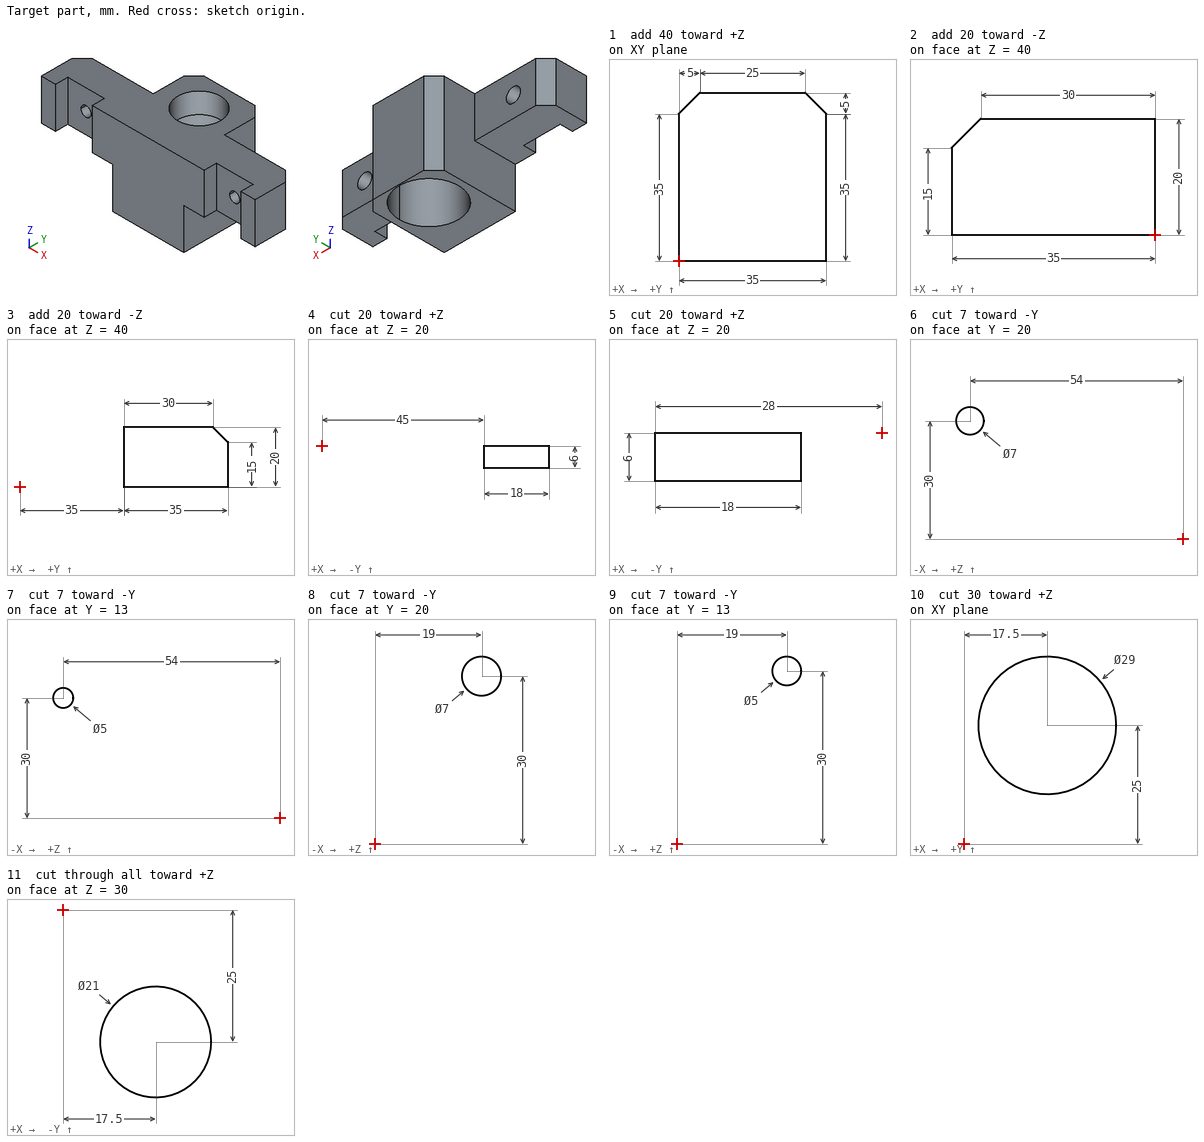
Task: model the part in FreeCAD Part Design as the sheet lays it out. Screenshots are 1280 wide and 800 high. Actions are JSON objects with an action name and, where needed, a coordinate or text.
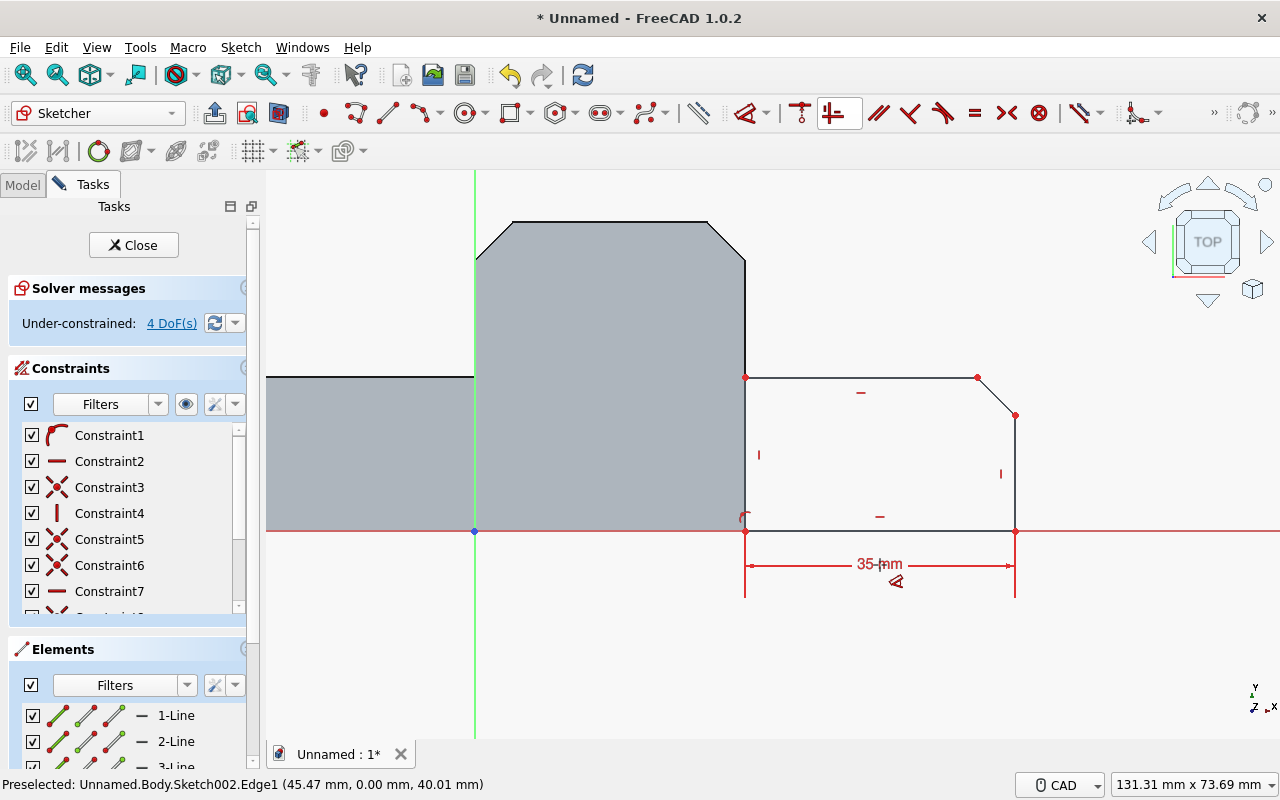
{"action": "left_click", "coordinate": [1015, 497]}
{"action": "left_click", "coordinate": [1049, 474]}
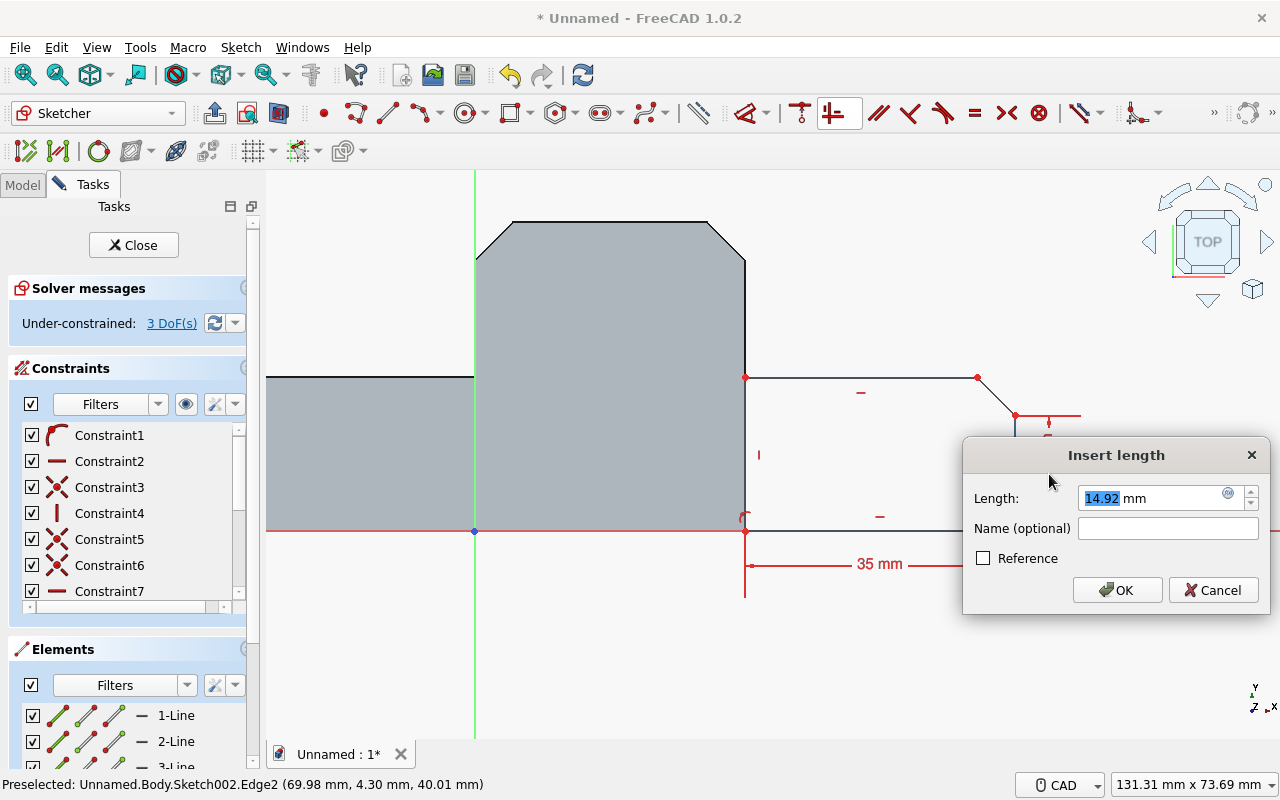
{"action": "type", "text": "15"}
{"action": "key", "text": "Return"}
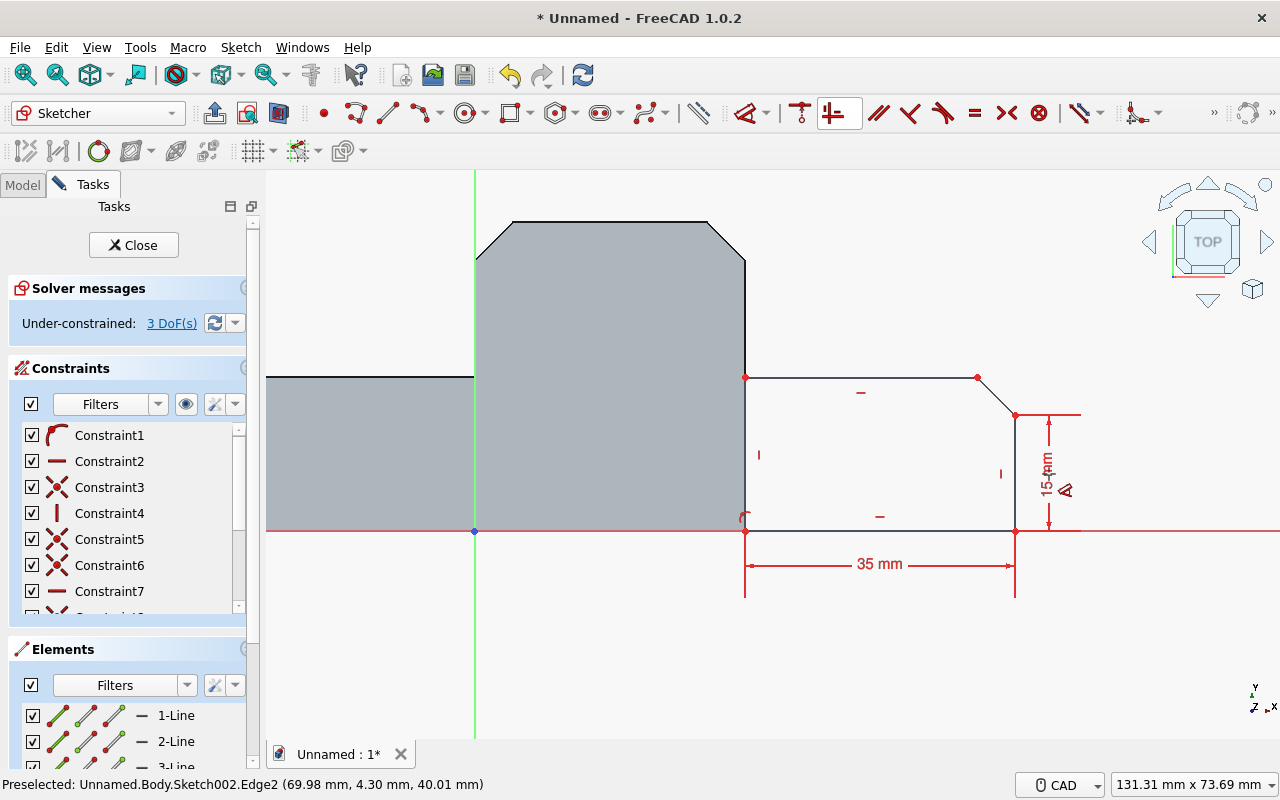
{"action": "left_click", "coordinate": [907, 378]}
{"action": "left_click", "coordinate": [861, 344]}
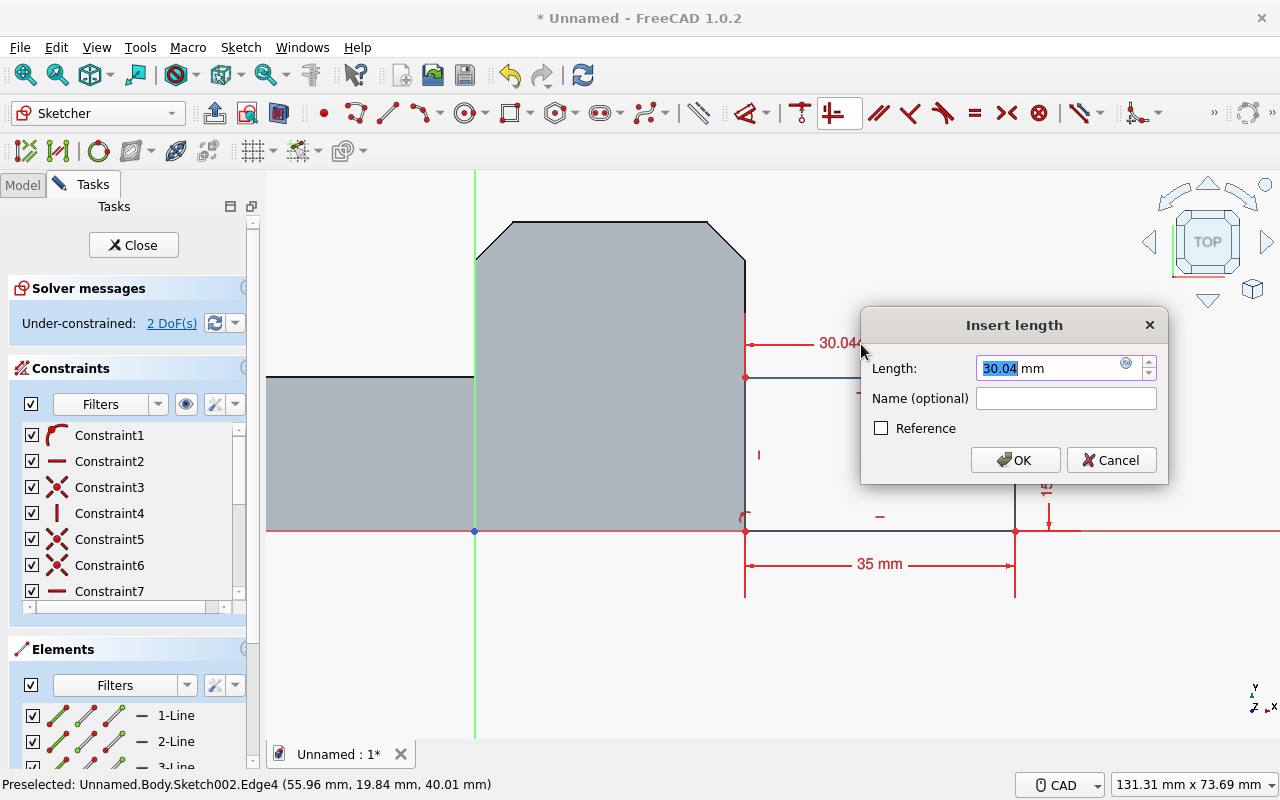
{"action": "type", "text": "30"}
{"action": "key", "text": "Return"}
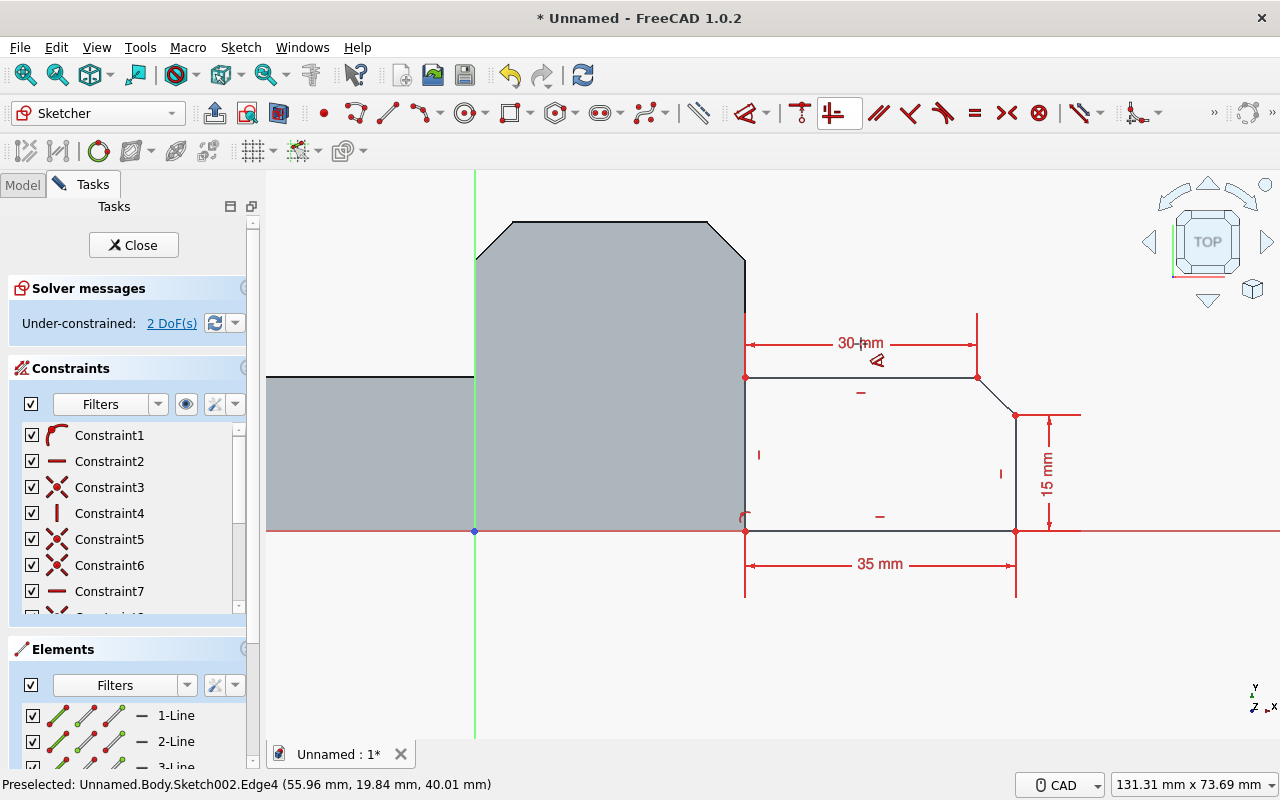
{"action": "left_click", "coordinate": [745, 424]}
{"action": "left_click", "coordinate": [779, 455]}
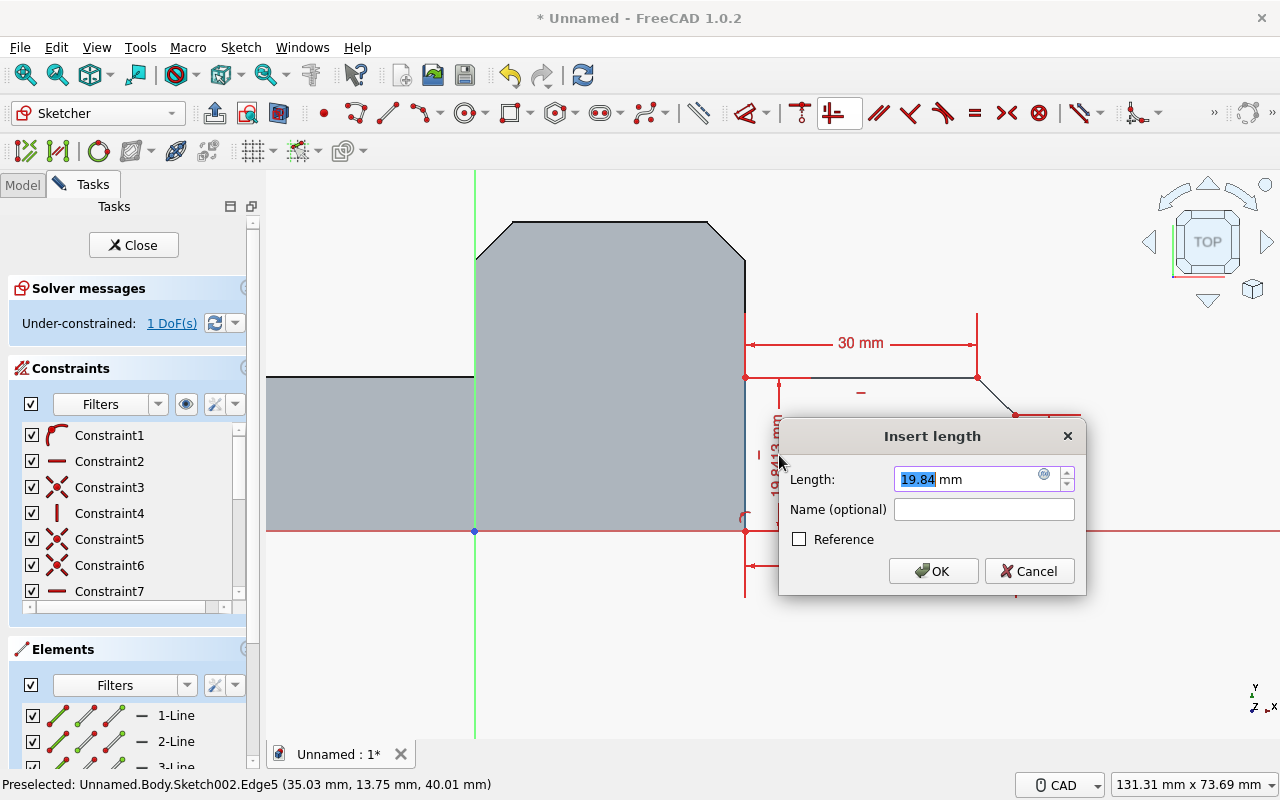
{"action": "type", "text": "20"}
{"action": "key", "text": "Return"}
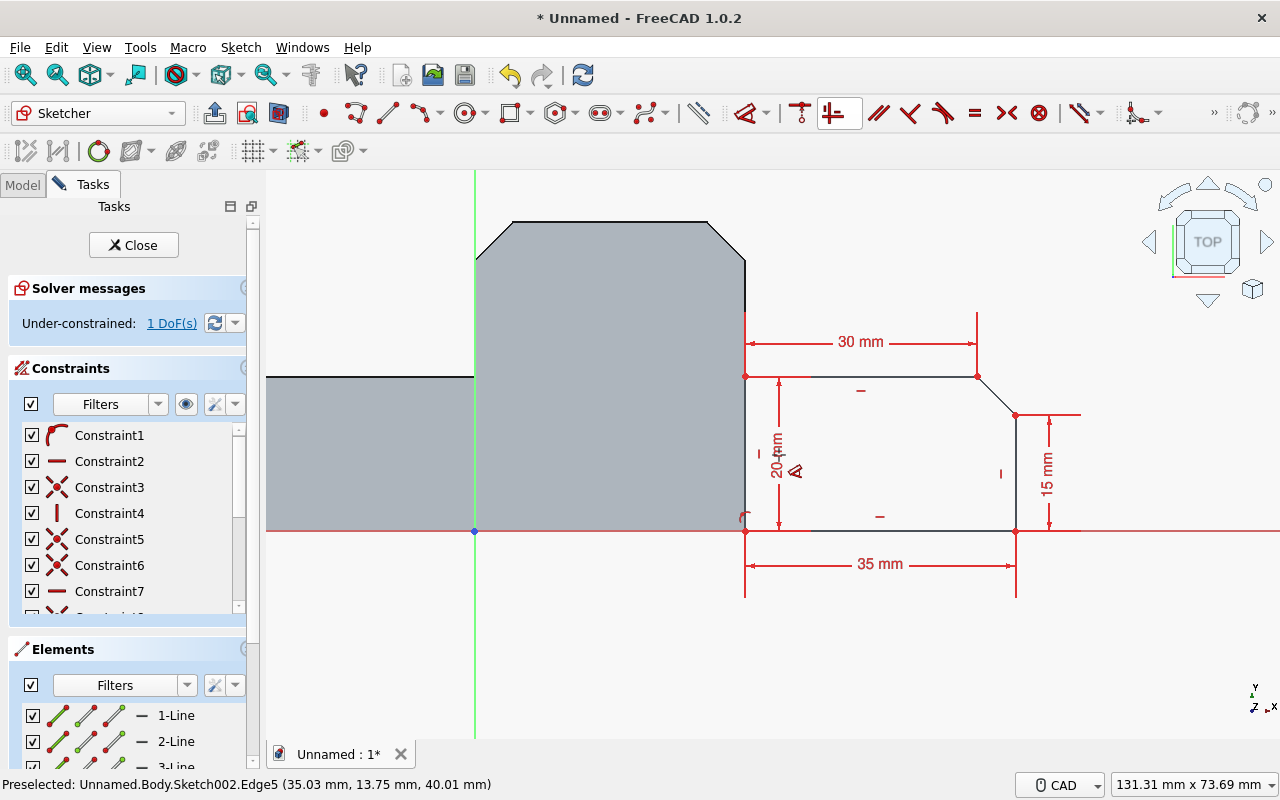
{"action": "left_click", "coordinate": [745, 531]}
{"action": "left_click", "coordinate": [610, 565]}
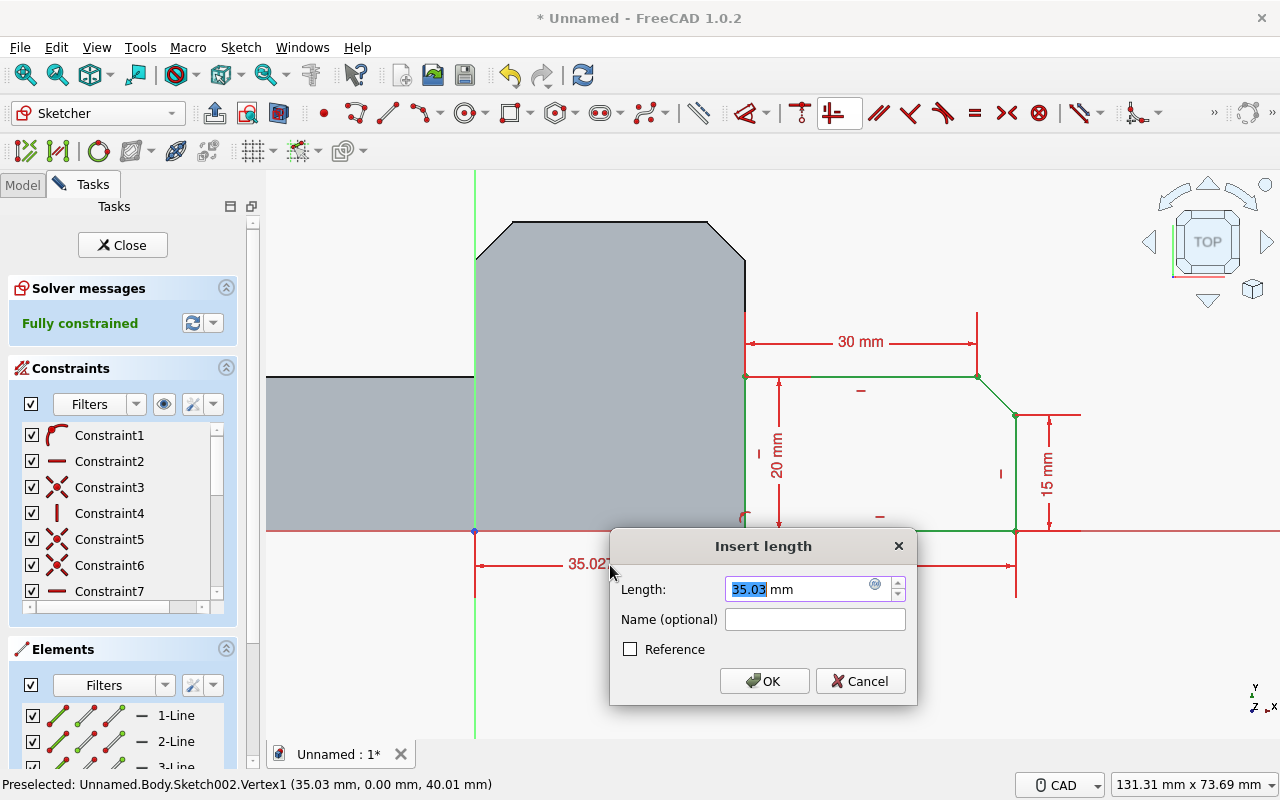
{"action": "type", "text": "35"}
{"action": "key", "text": "Return"}
{"action": "key", "text": "Escape"}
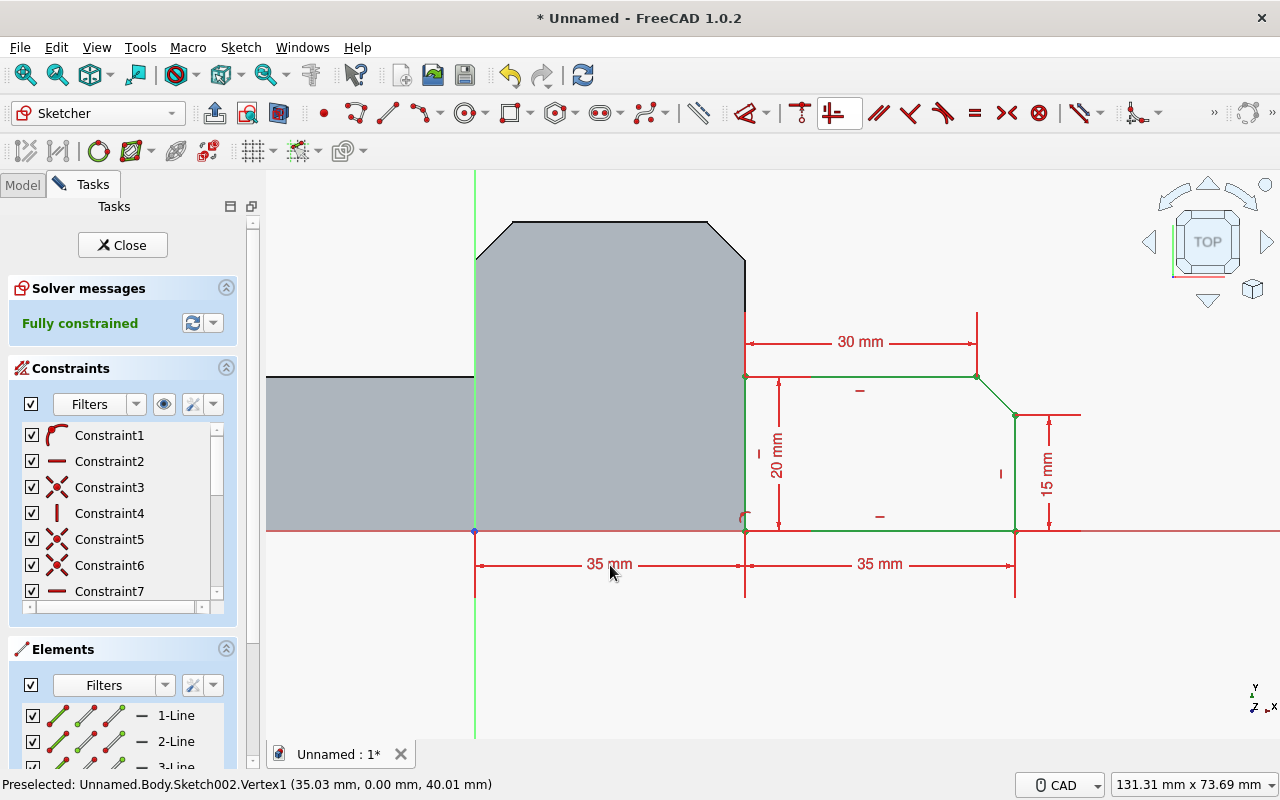
{"action": "left_click", "coordinate": [123, 245]}